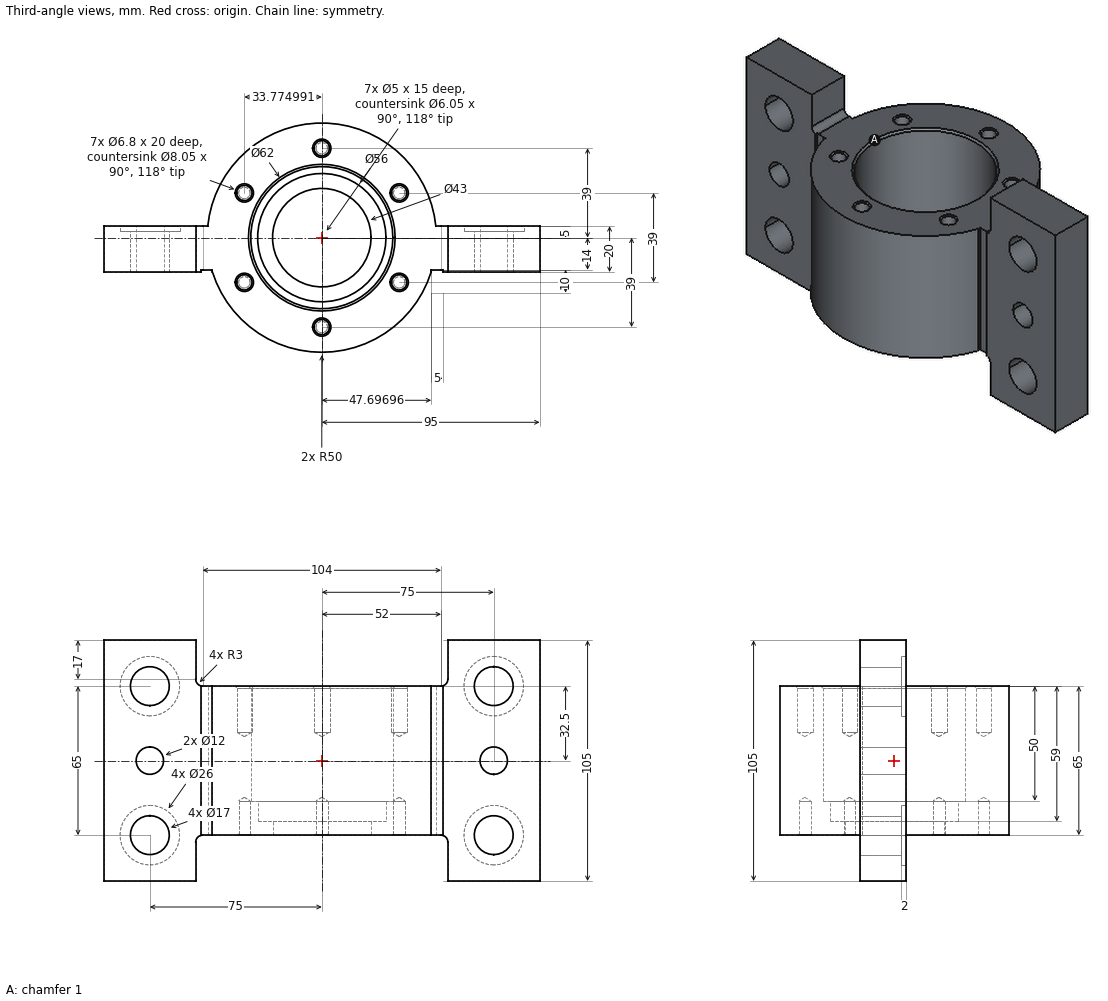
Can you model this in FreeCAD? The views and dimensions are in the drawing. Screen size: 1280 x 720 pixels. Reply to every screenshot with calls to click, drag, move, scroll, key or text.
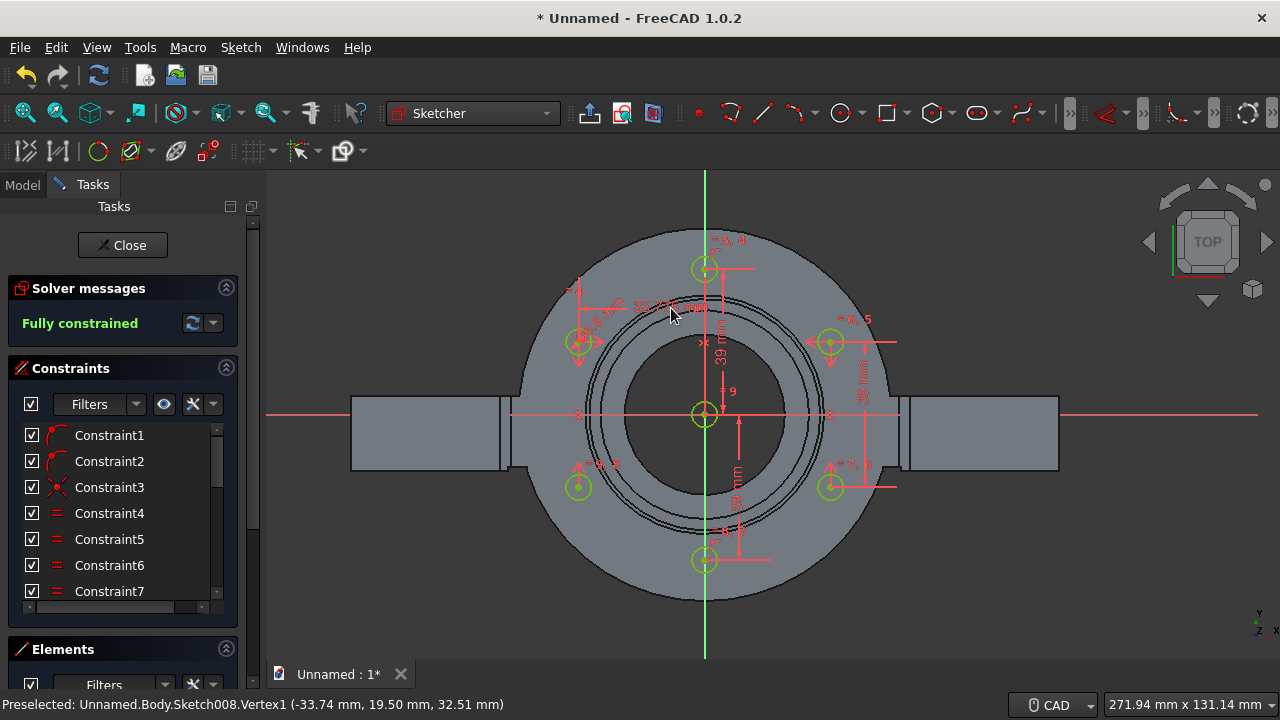
click(123, 245)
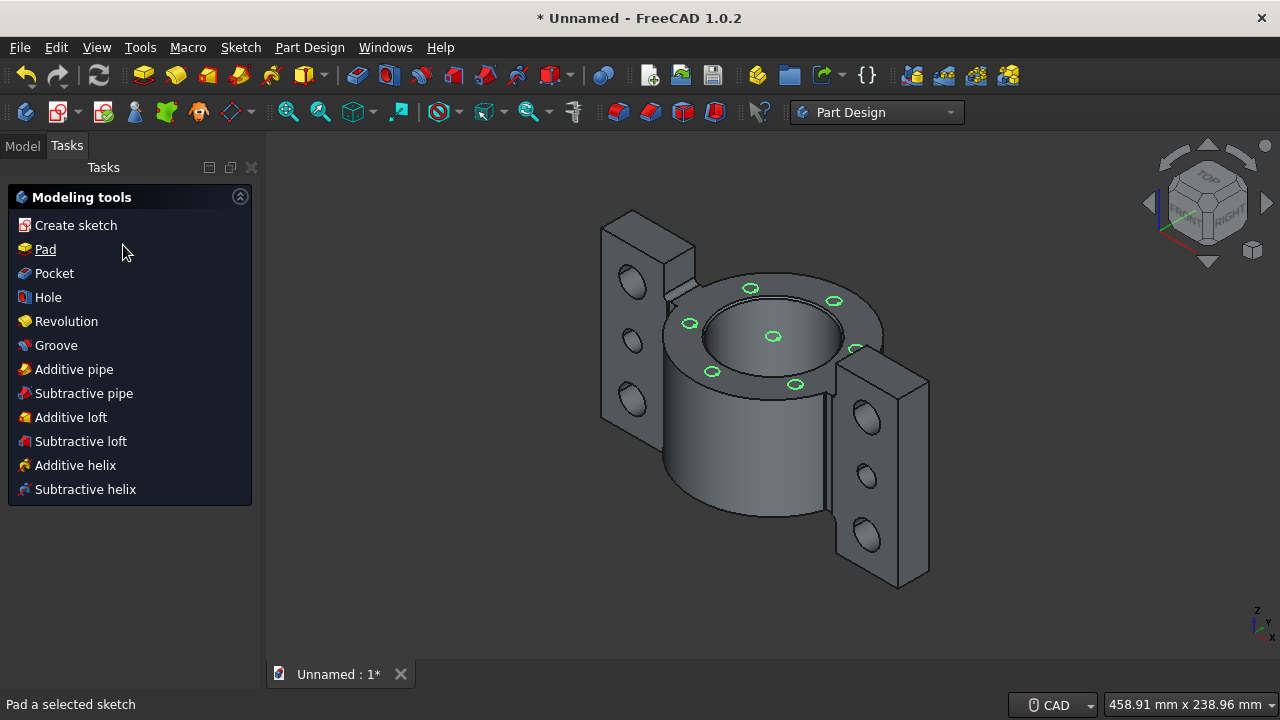
click(390, 76)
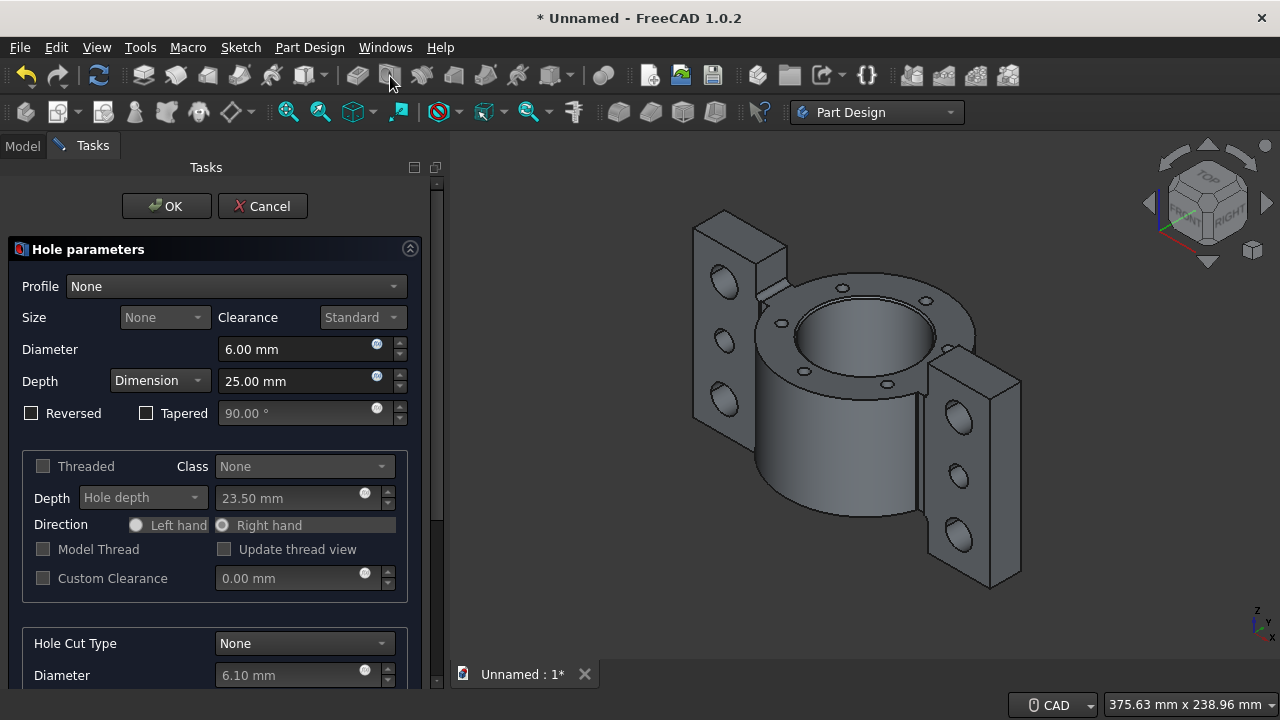
triple_click(305, 349)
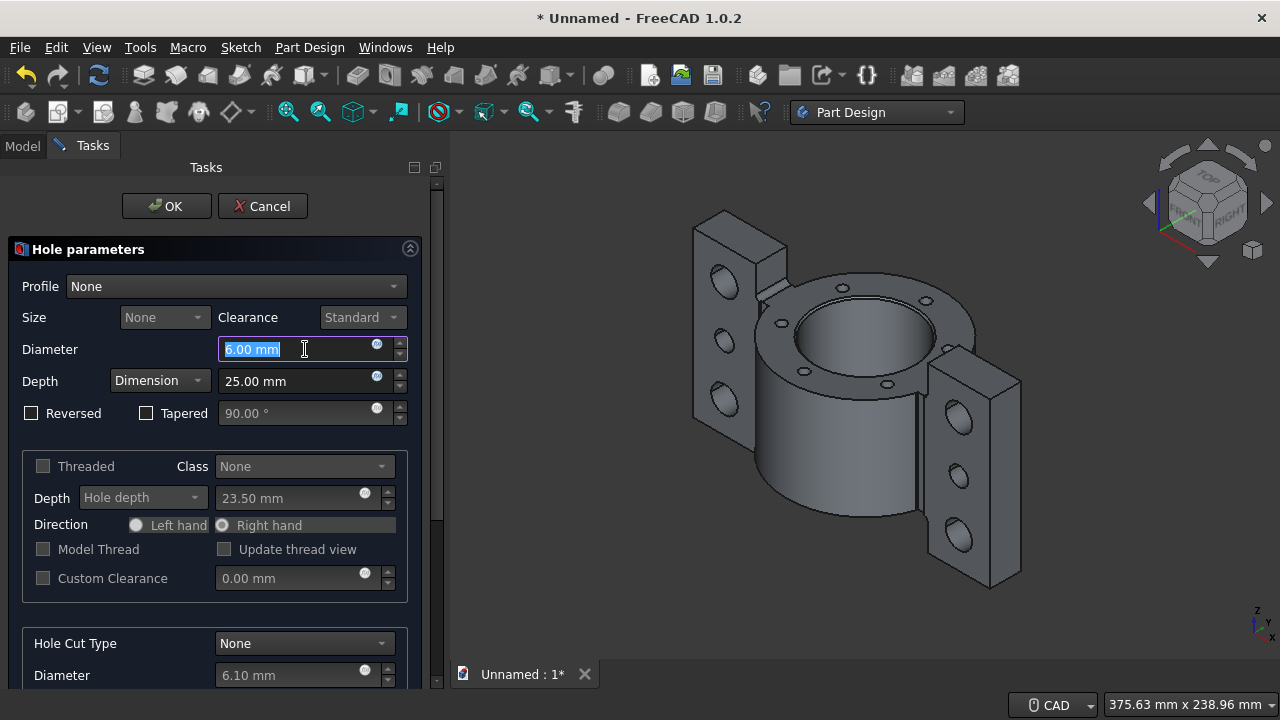
text(6.8)
key(Tab)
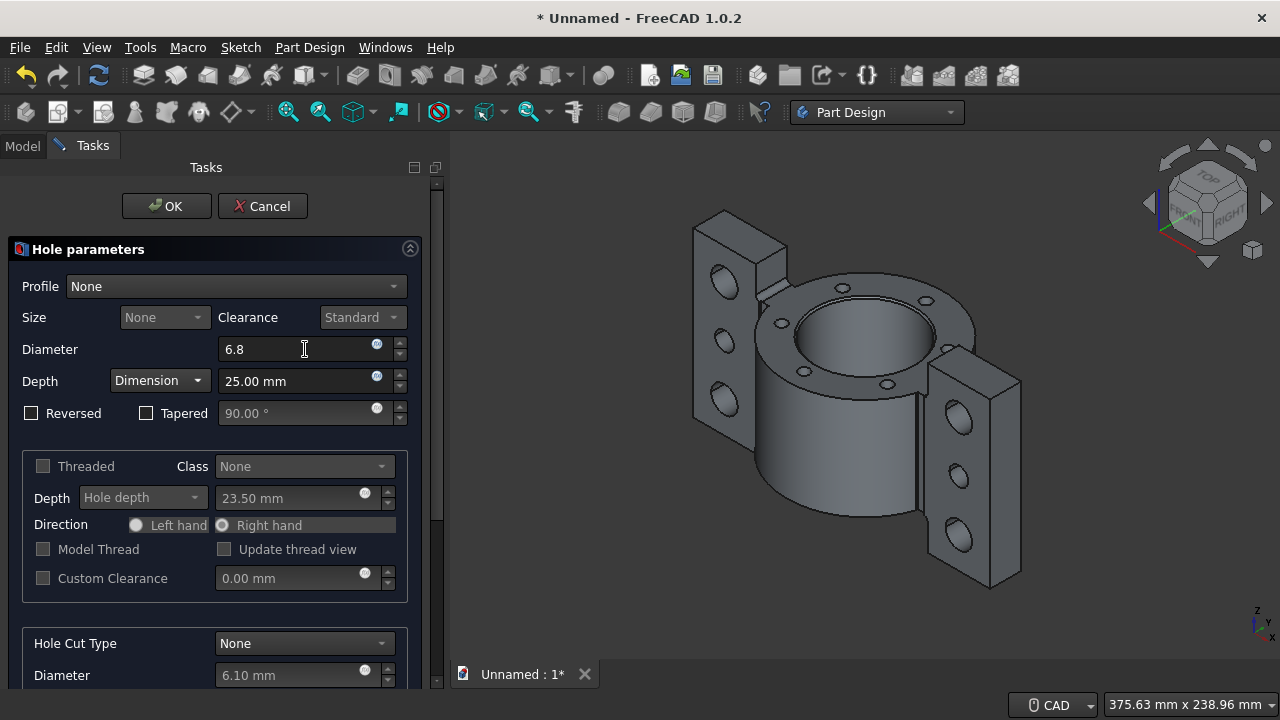
triple_click(305, 381)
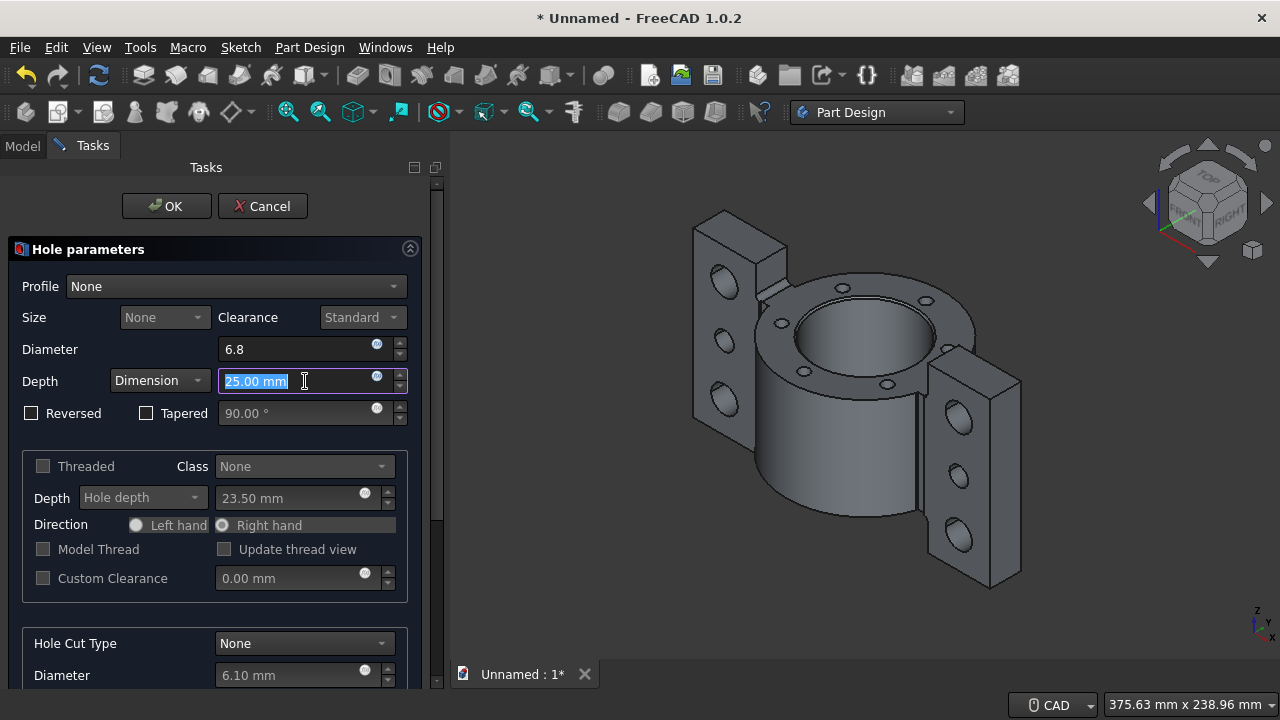
text(20)
key(Tab)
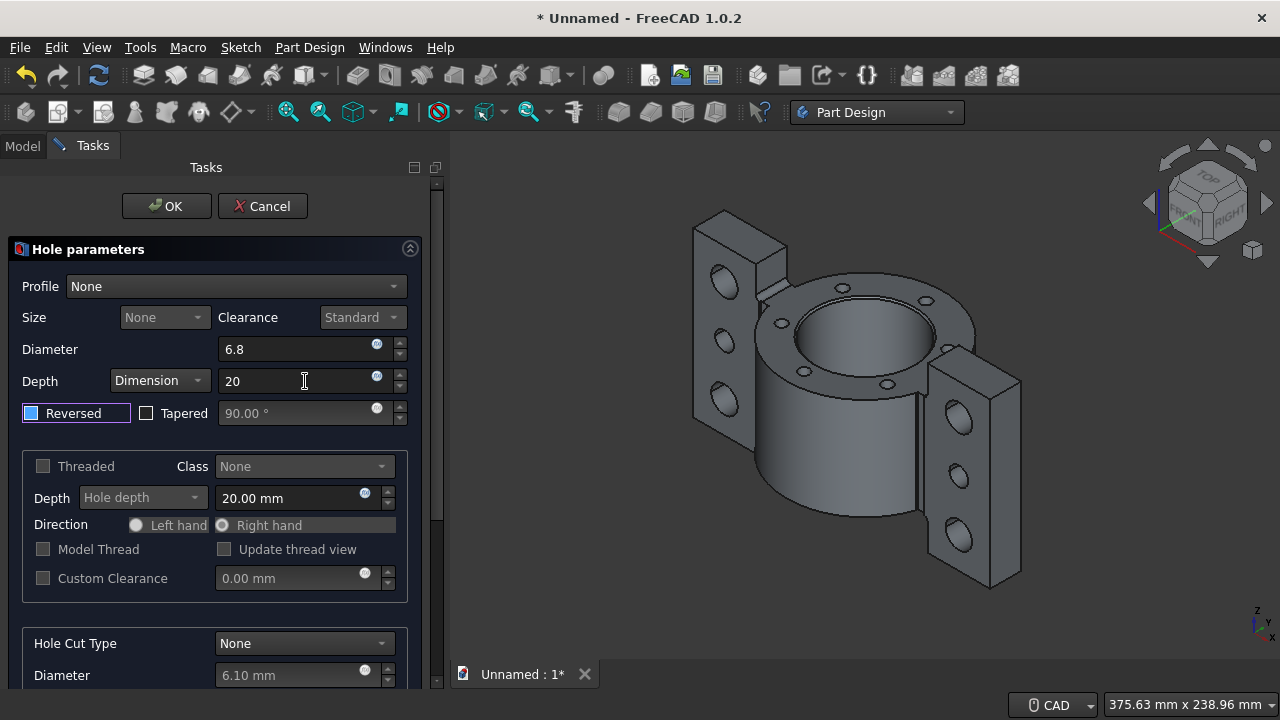
click(306, 644)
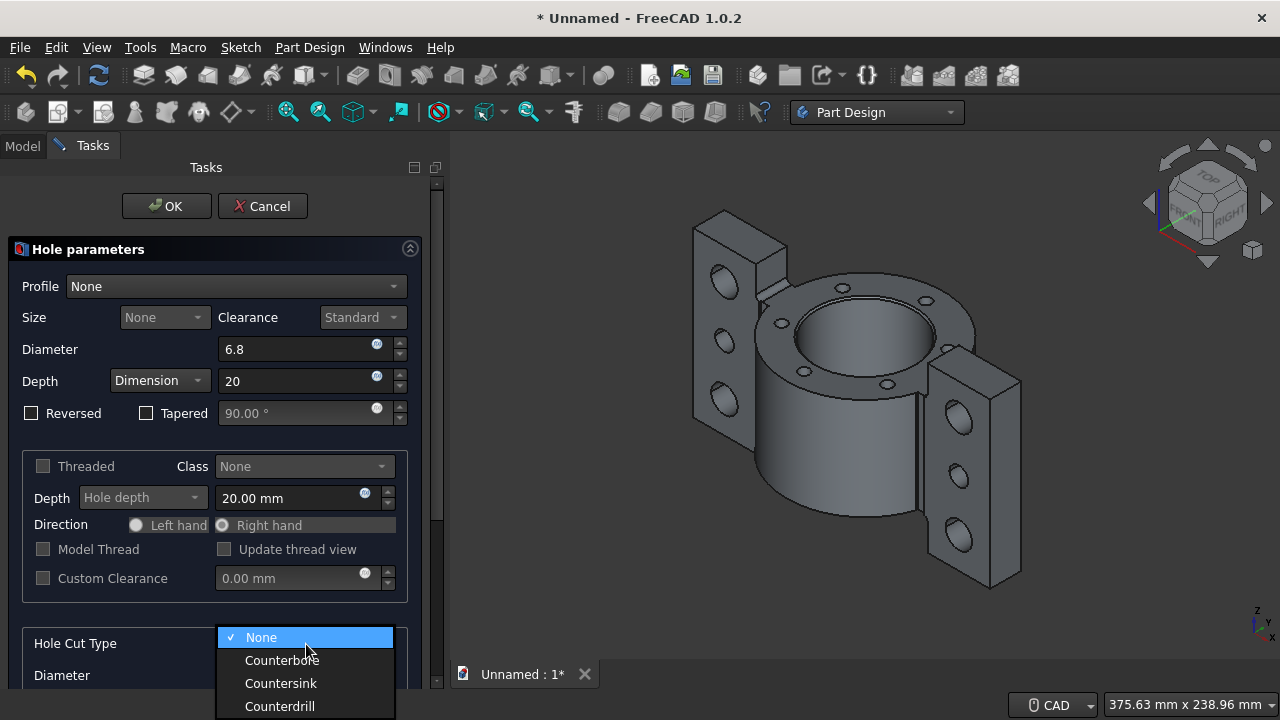
click(304, 684)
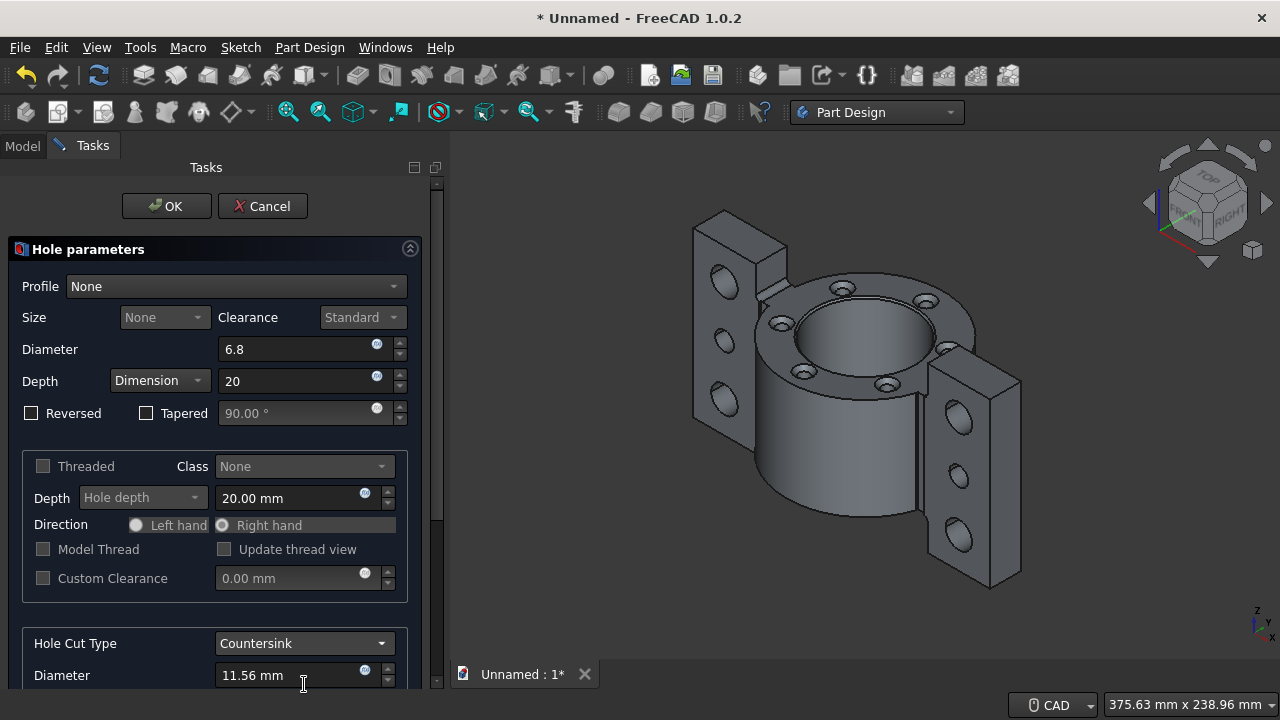
triple_click(298, 675)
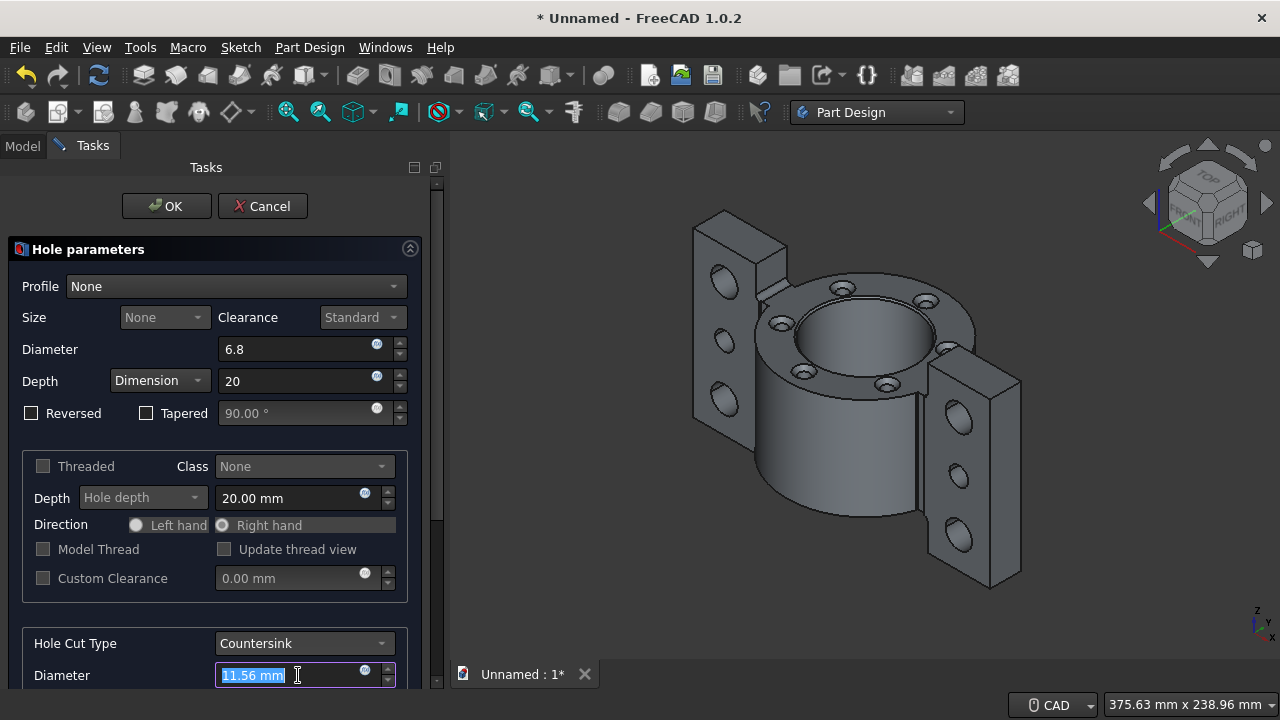
text(8.05)
key(Tab)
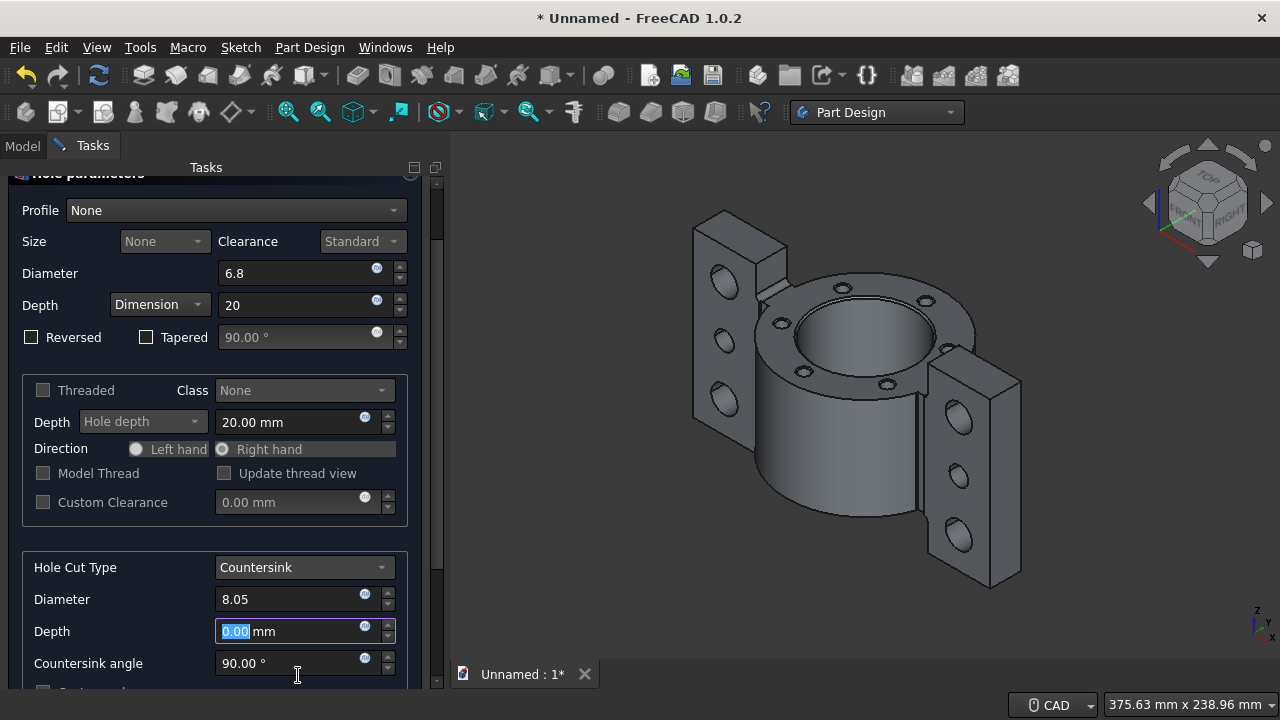
scroll(437, 432, up, 3)